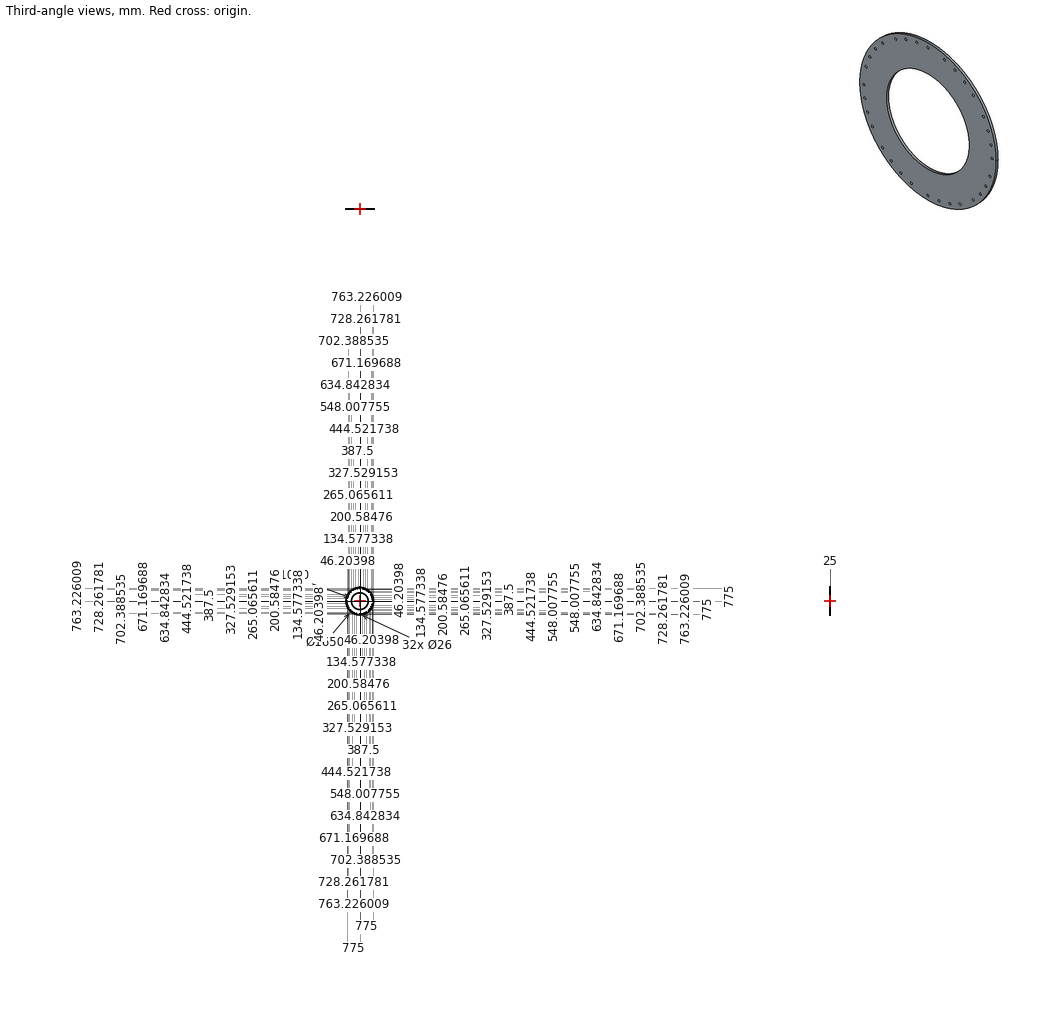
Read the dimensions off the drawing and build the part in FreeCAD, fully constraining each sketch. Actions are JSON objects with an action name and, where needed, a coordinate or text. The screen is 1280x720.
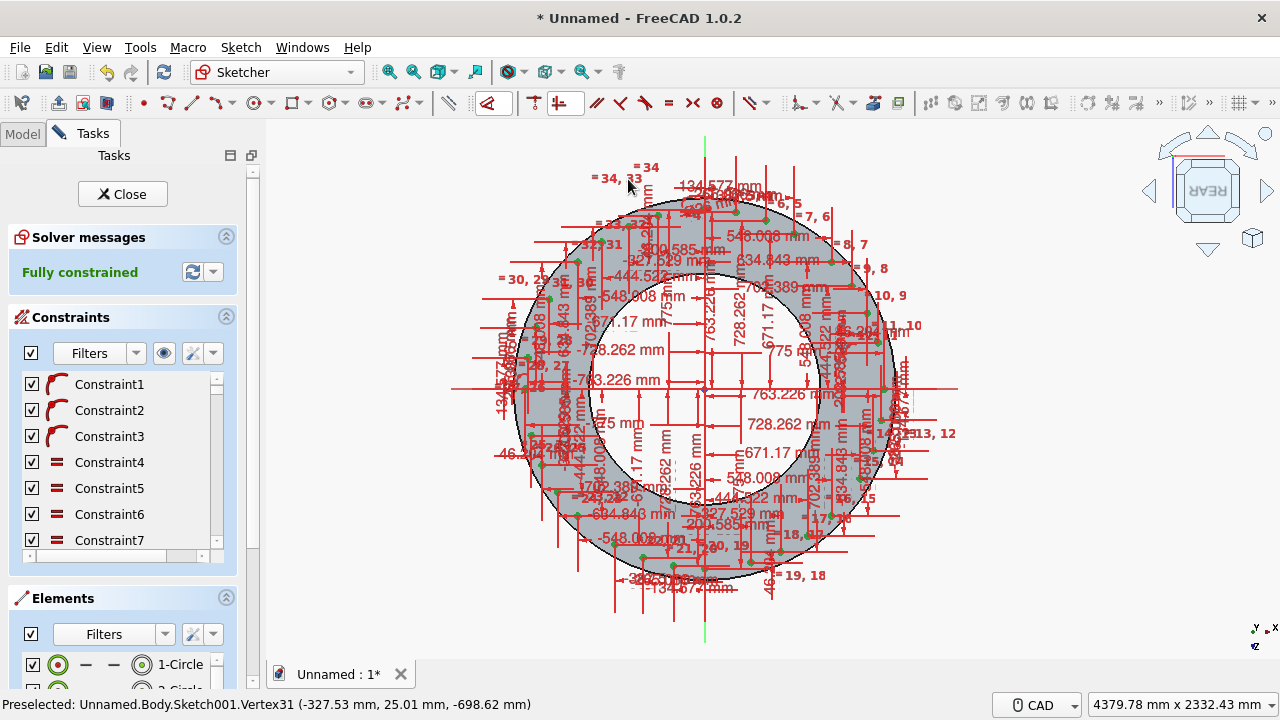
{"action": "left_click", "coordinate": [123, 194]}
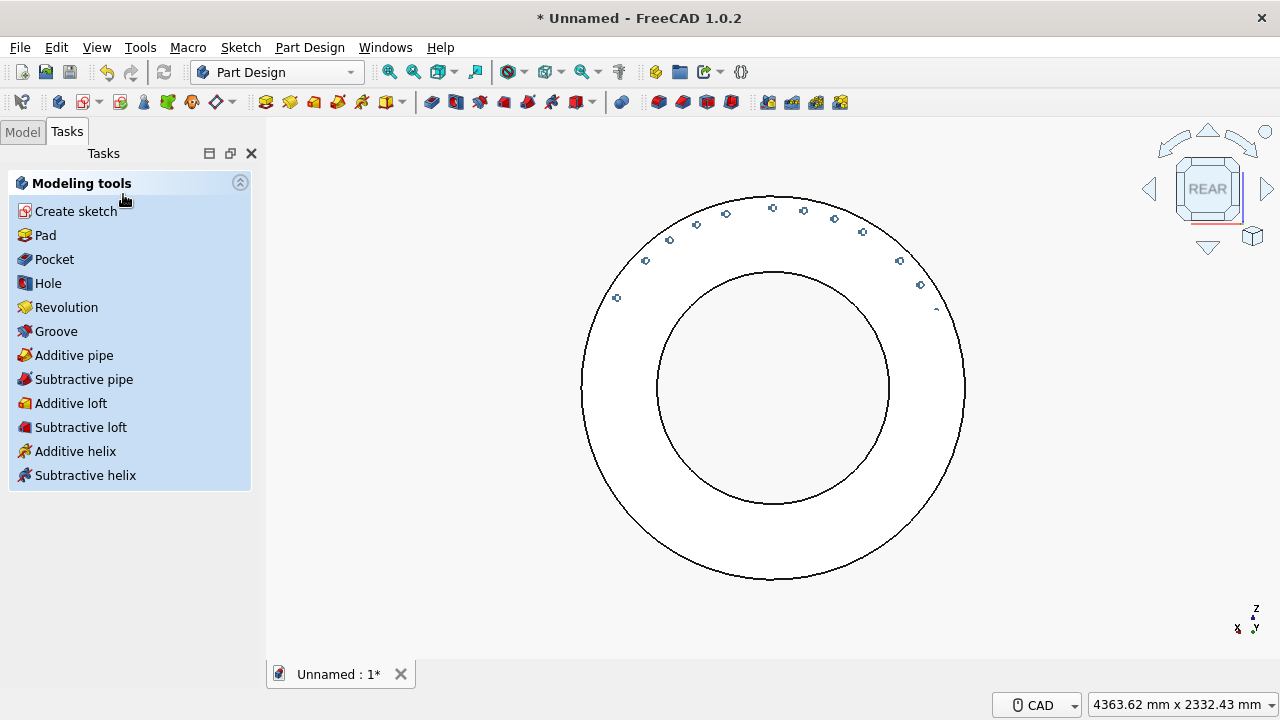
{"action": "left_click", "coordinate": [432, 102]}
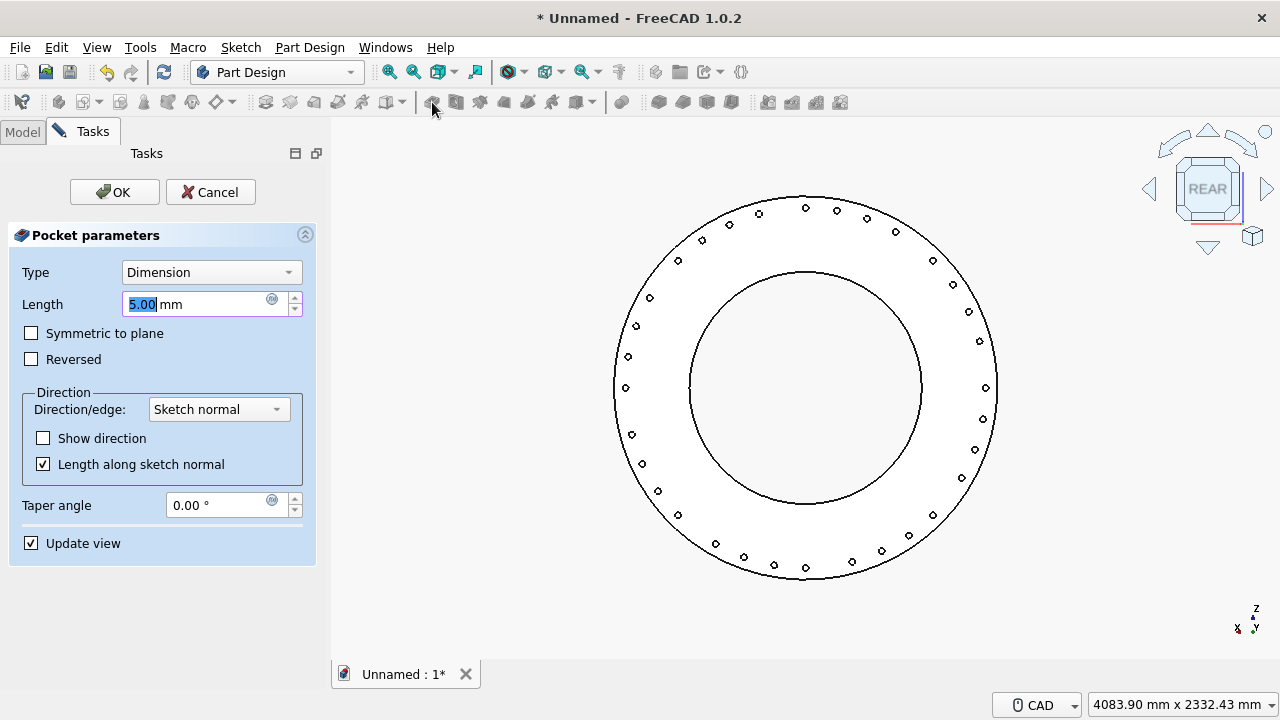
{"action": "left_click", "coordinate": [212, 272]}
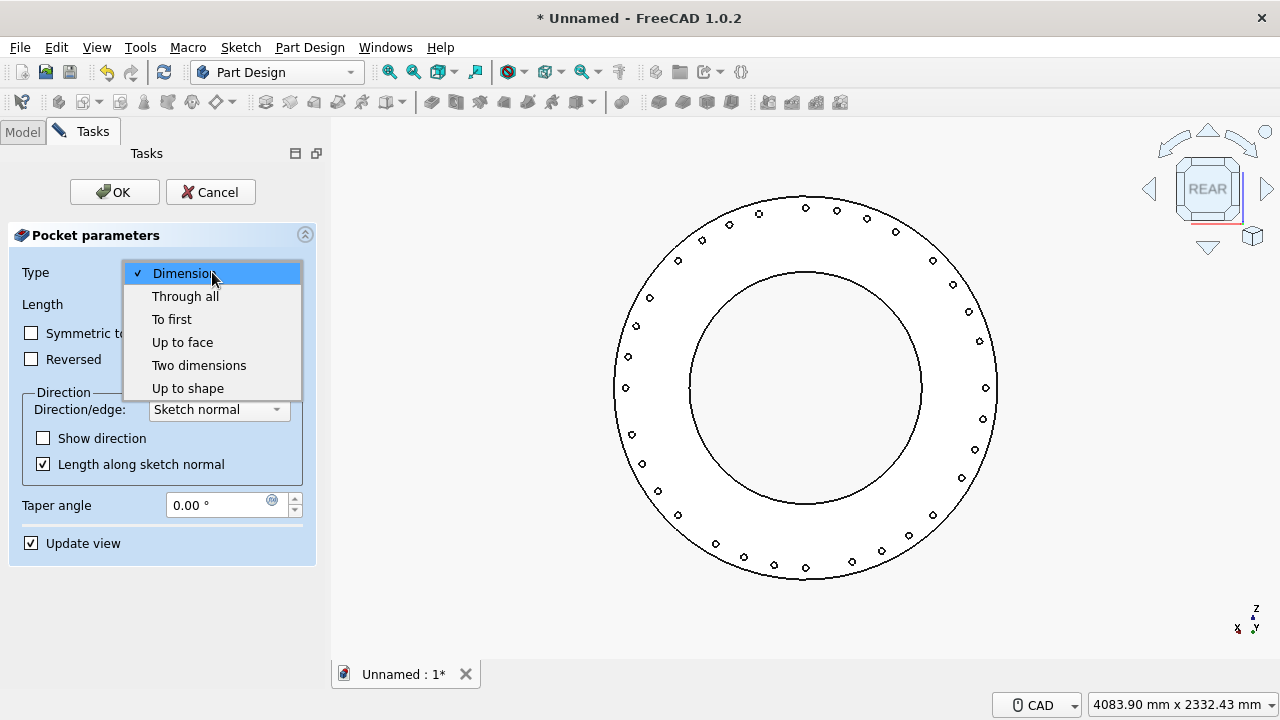
{"action": "left_click", "coordinate": [212, 296]}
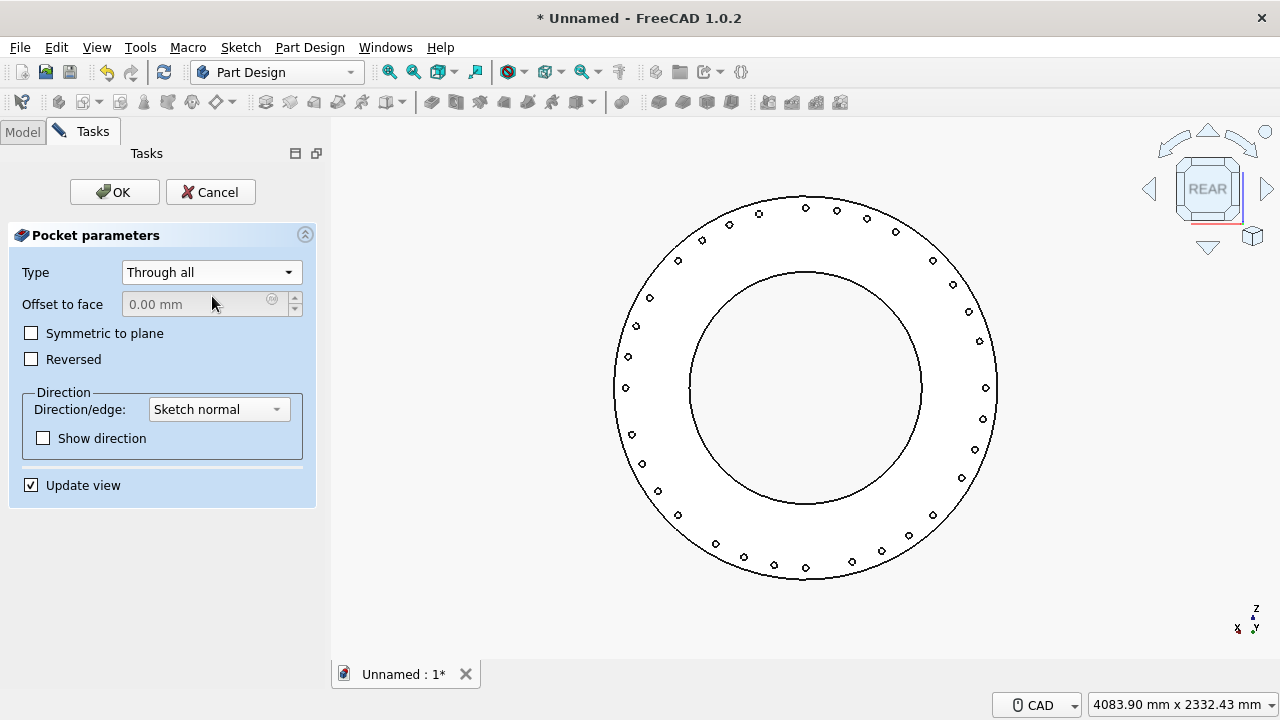
{"action": "left_click", "coordinate": [115, 192]}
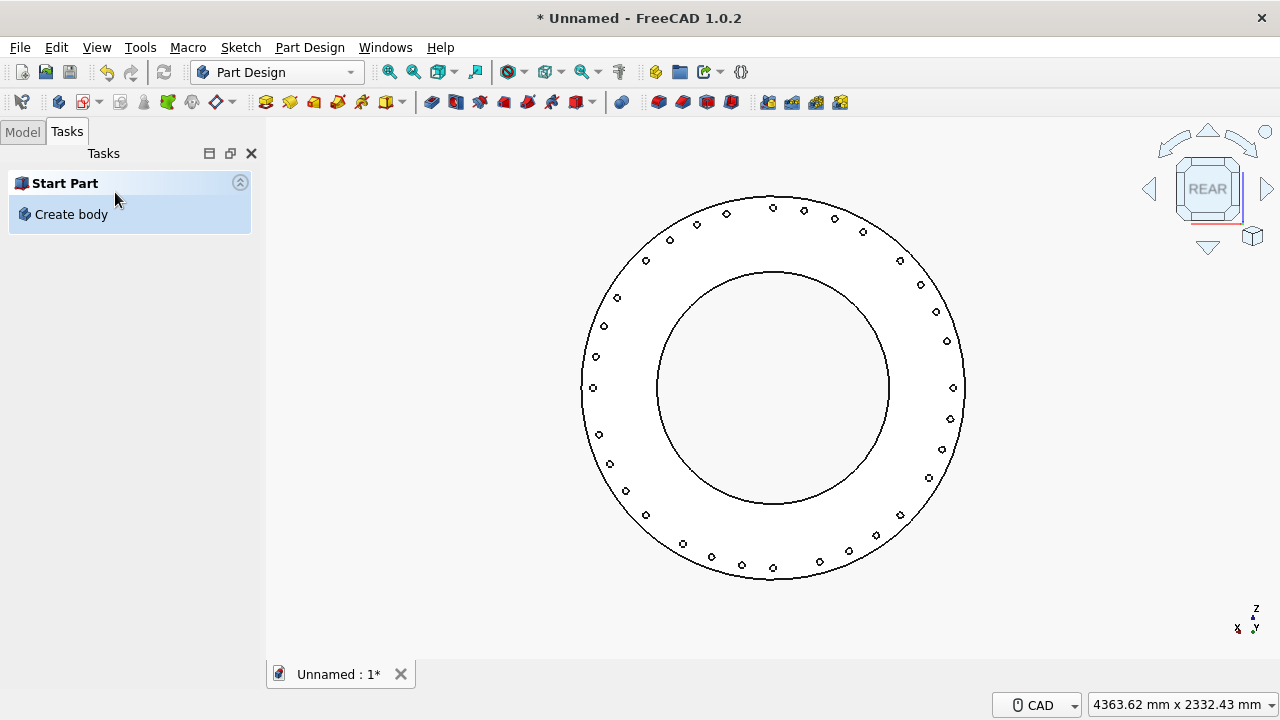
{"action": "key", "text": "0"}